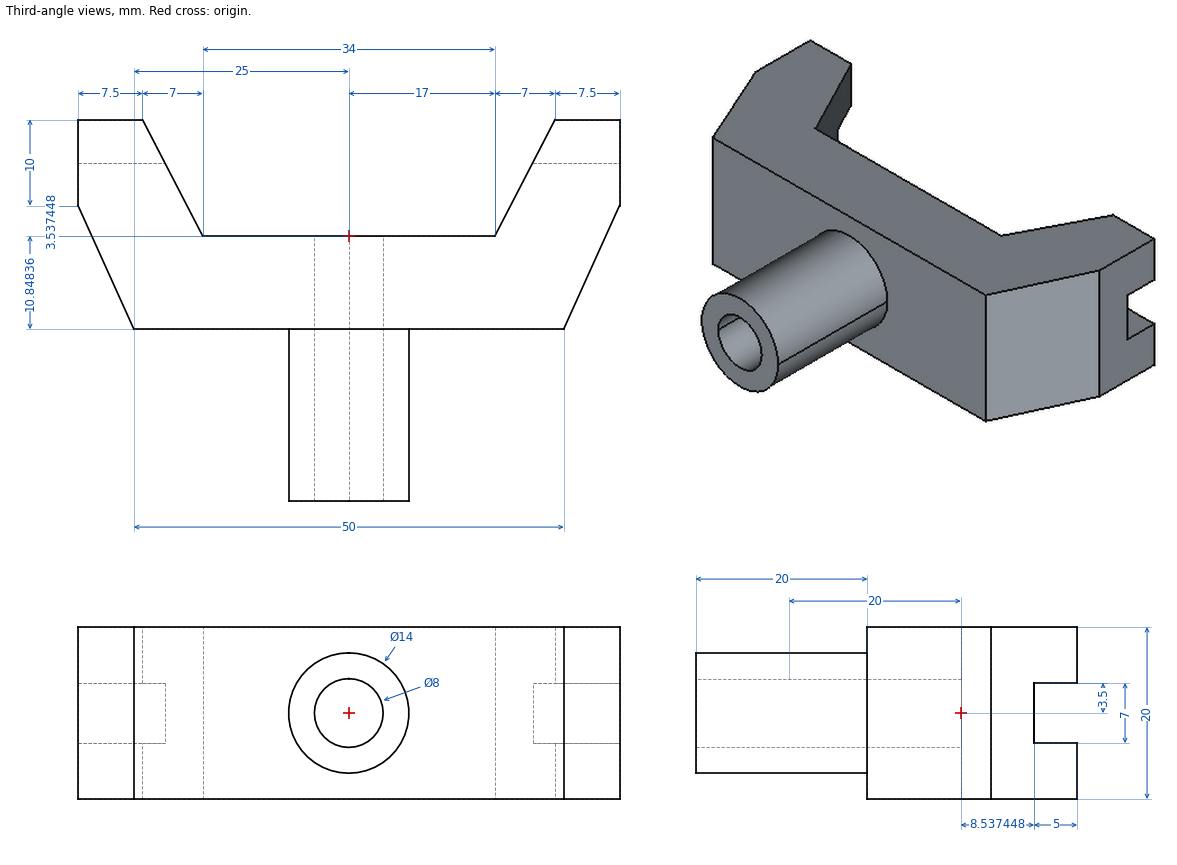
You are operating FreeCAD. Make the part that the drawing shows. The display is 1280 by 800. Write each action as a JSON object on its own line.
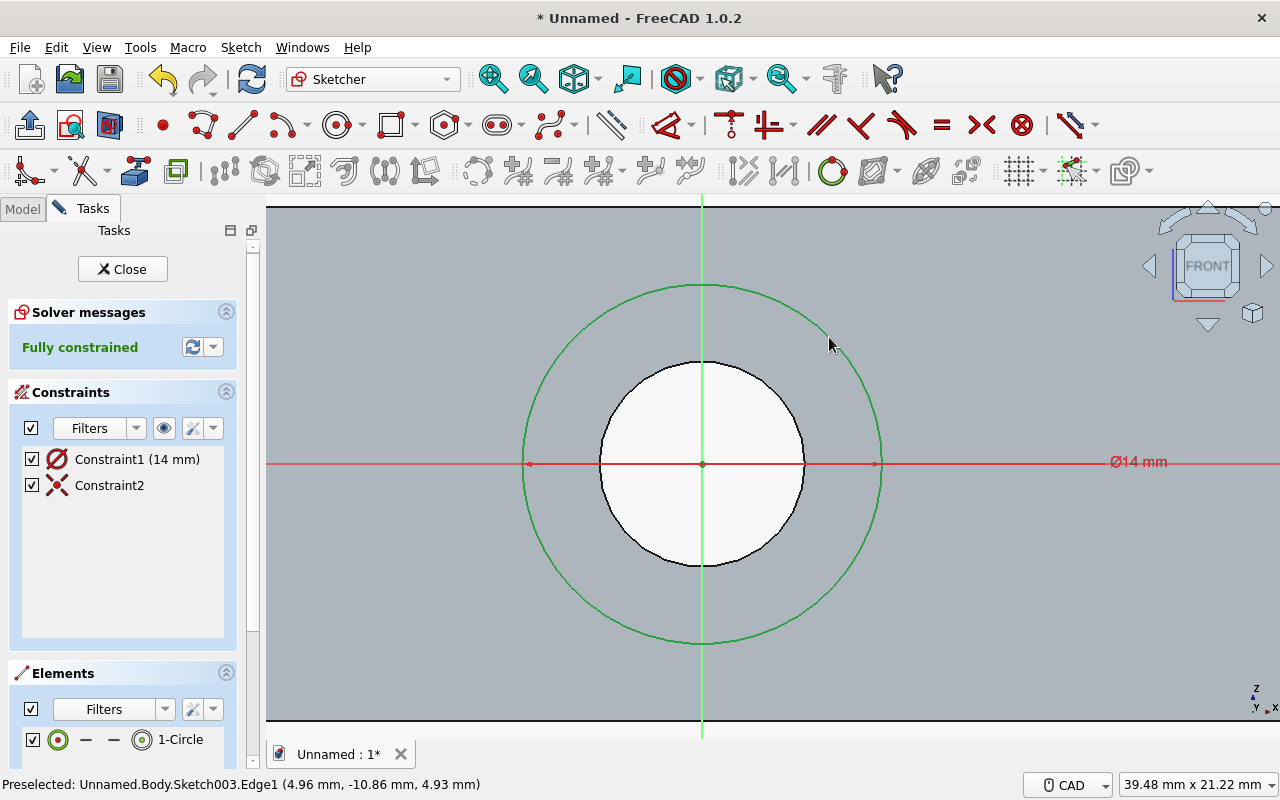
{"action": "left_click", "coordinate": [123, 269]}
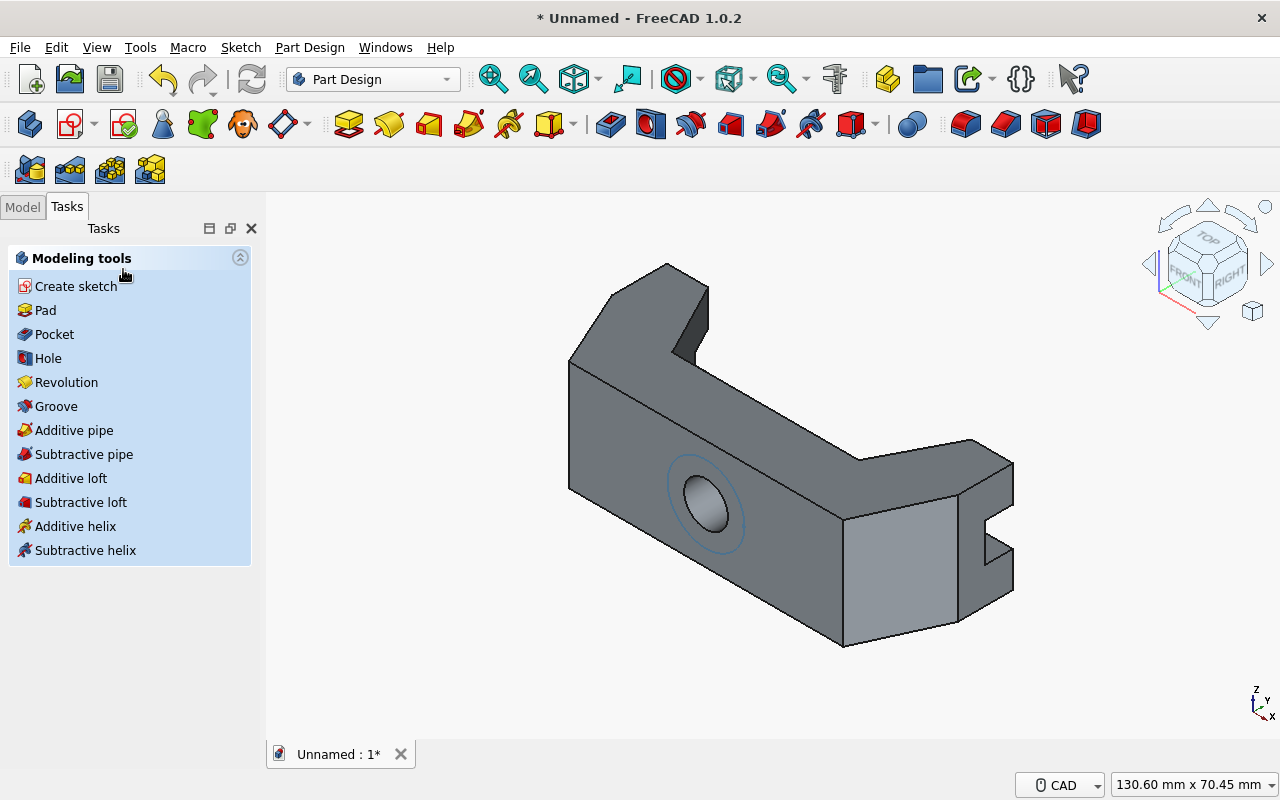
{"action": "left_click", "coordinate": [350, 124]}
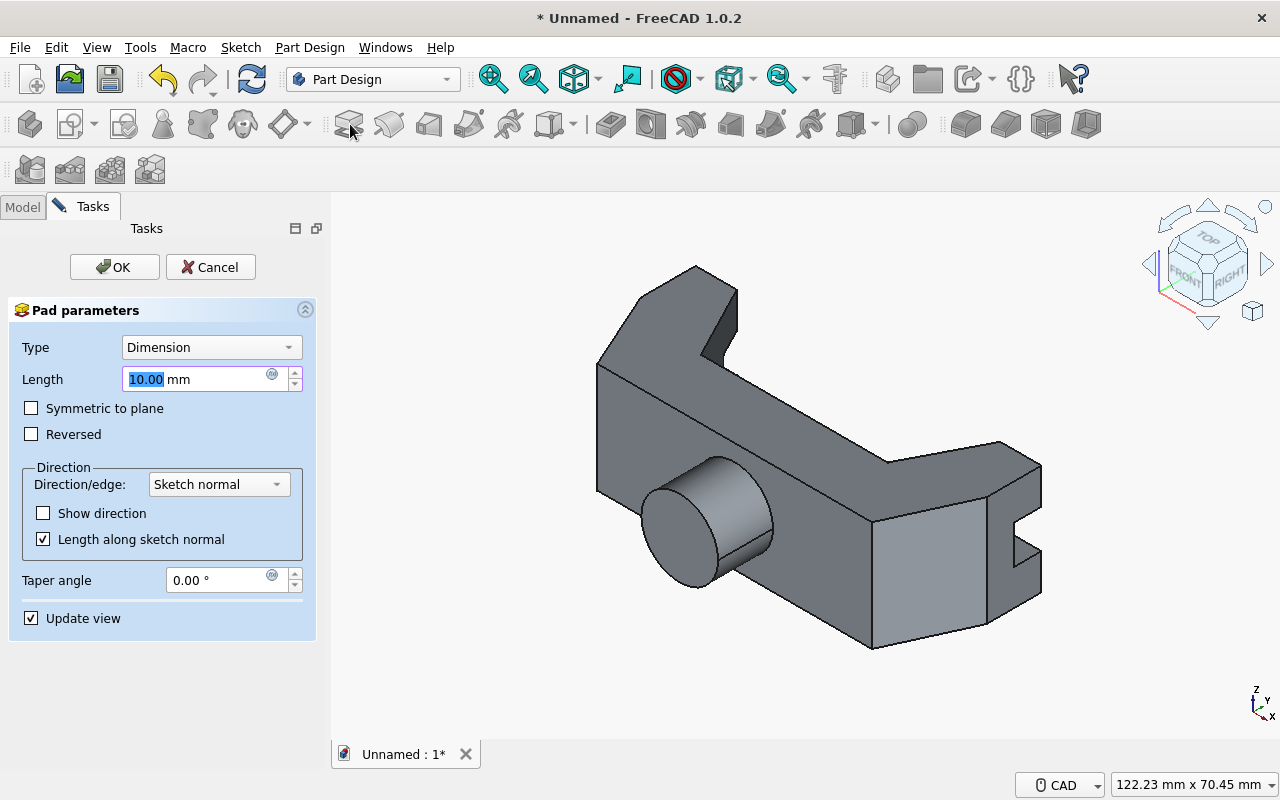
{"action": "type", "text": "20"}
{"action": "key", "text": "Tab"}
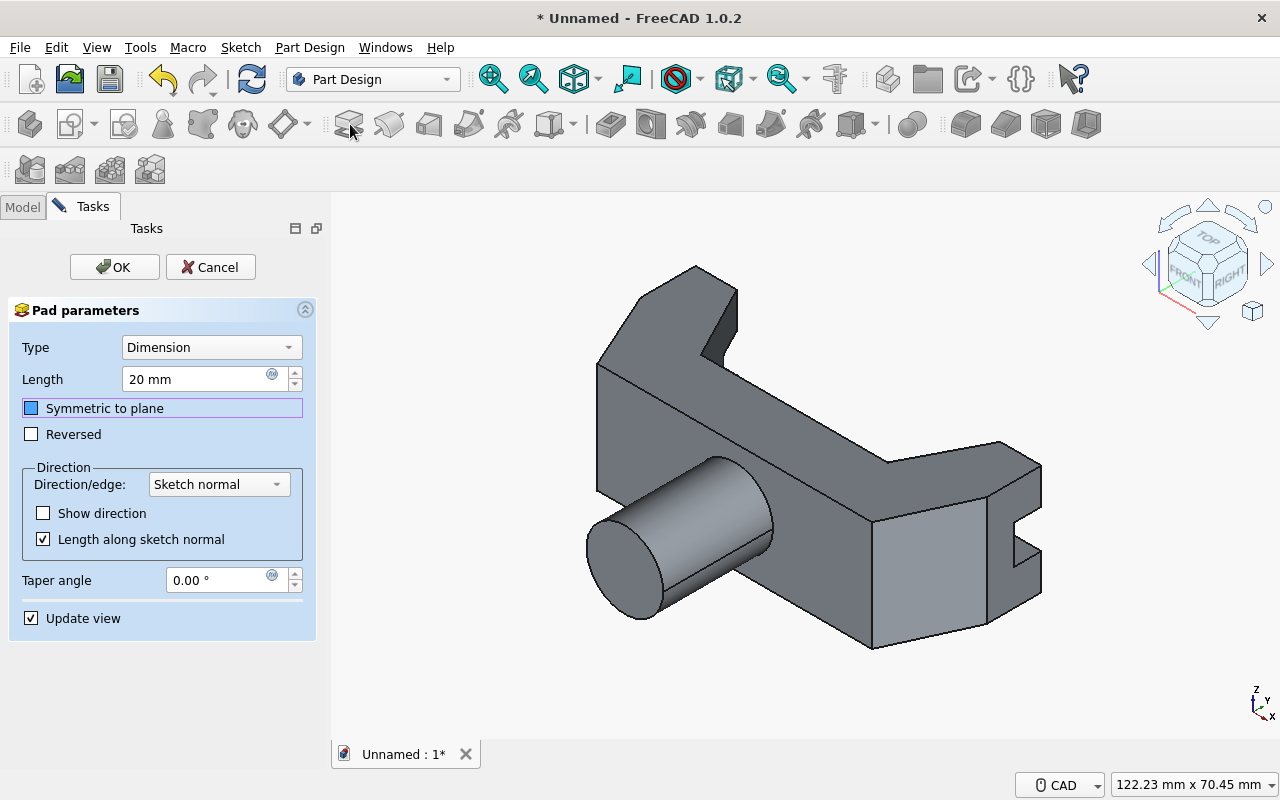
{"action": "left_click", "coordinate": [115, 267]}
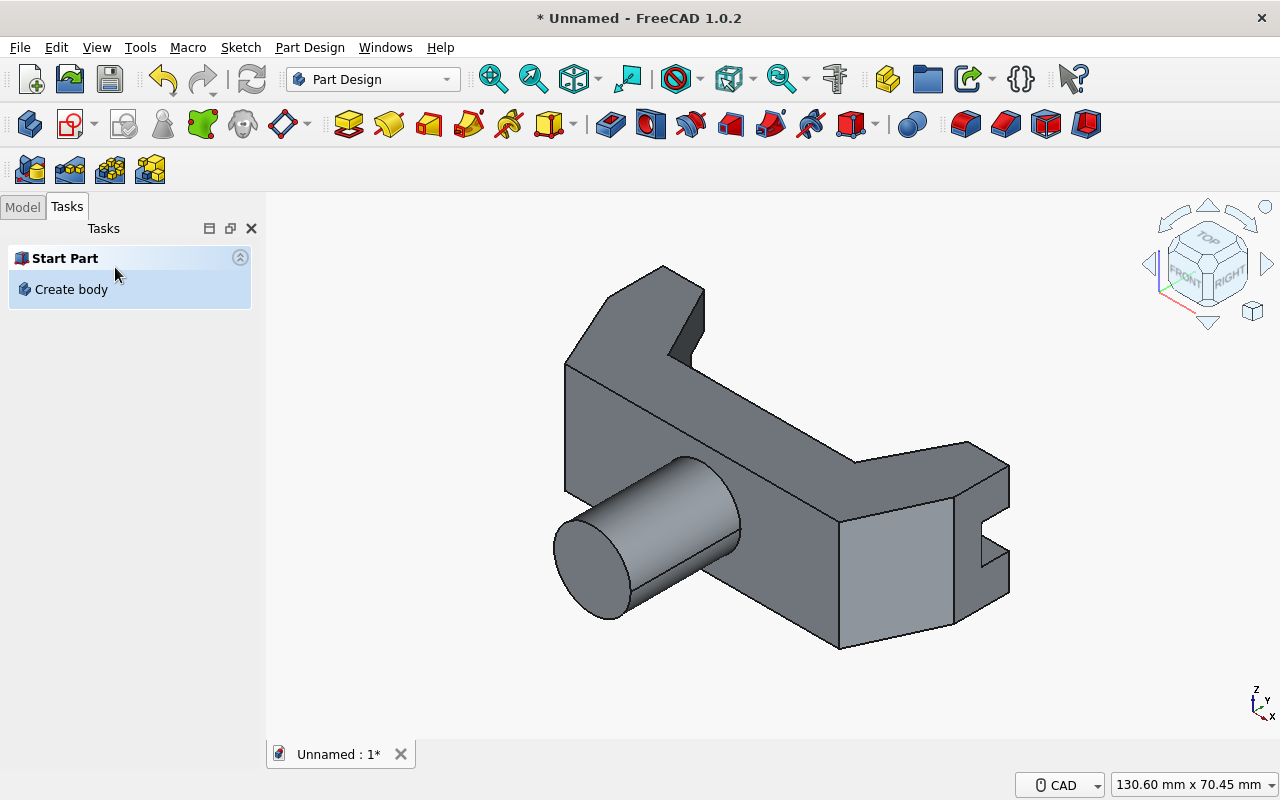
{"action": "key", "text": "4"}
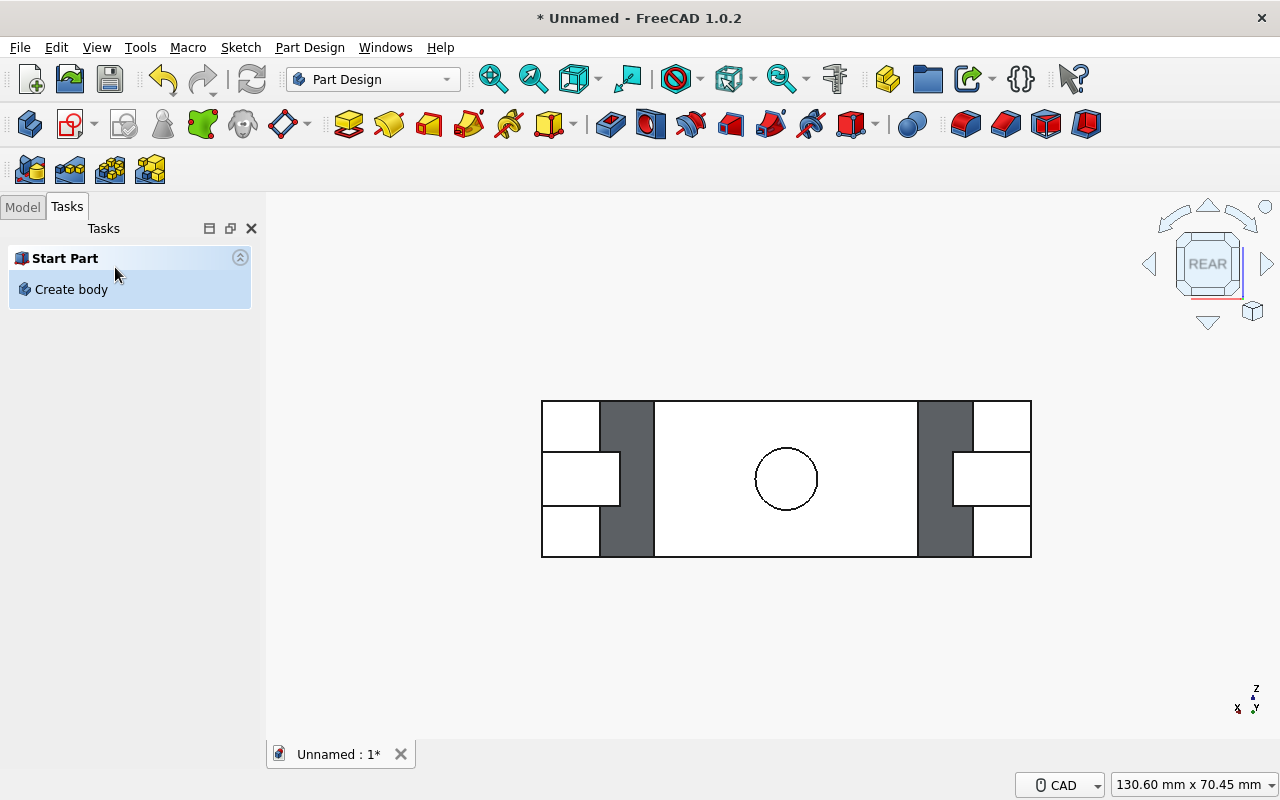
{"action": "left_click", "coordinate": [711, 500]}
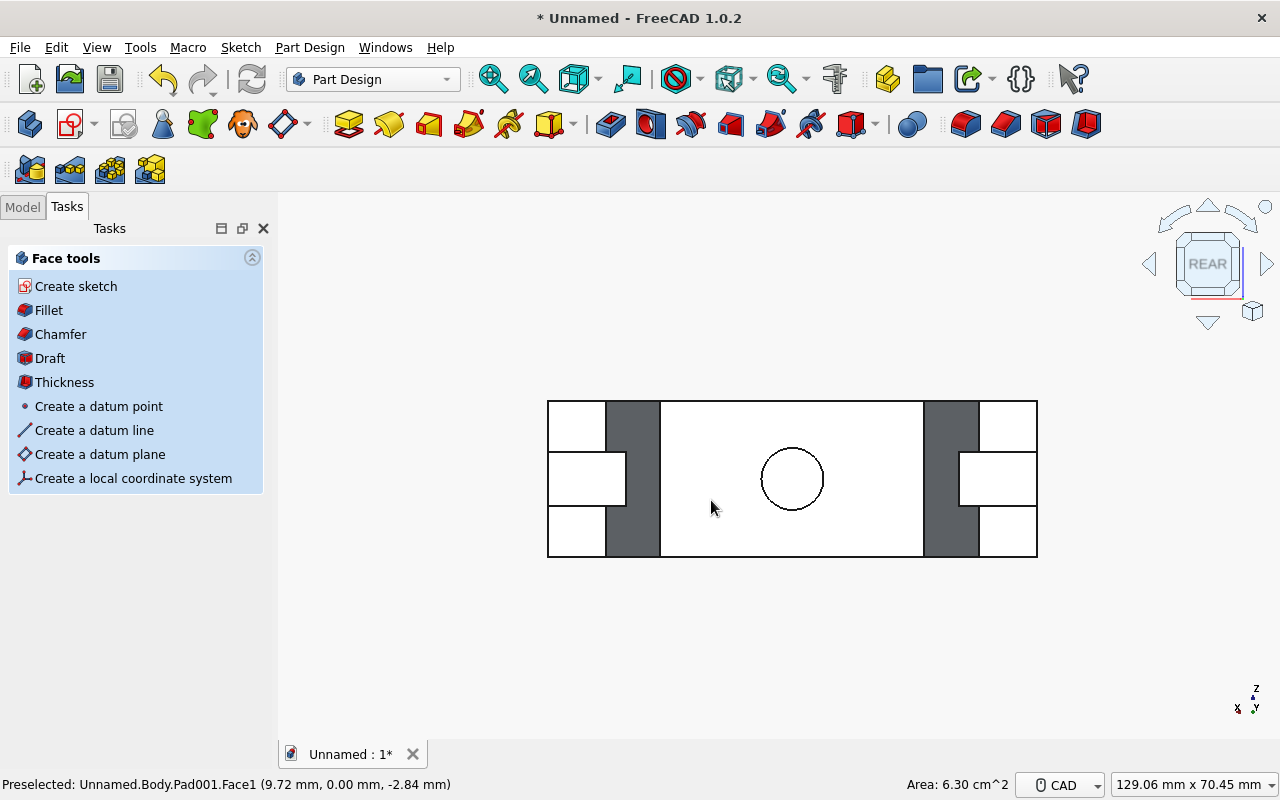
{"action": "left_click", "coordinate": [70, 124]}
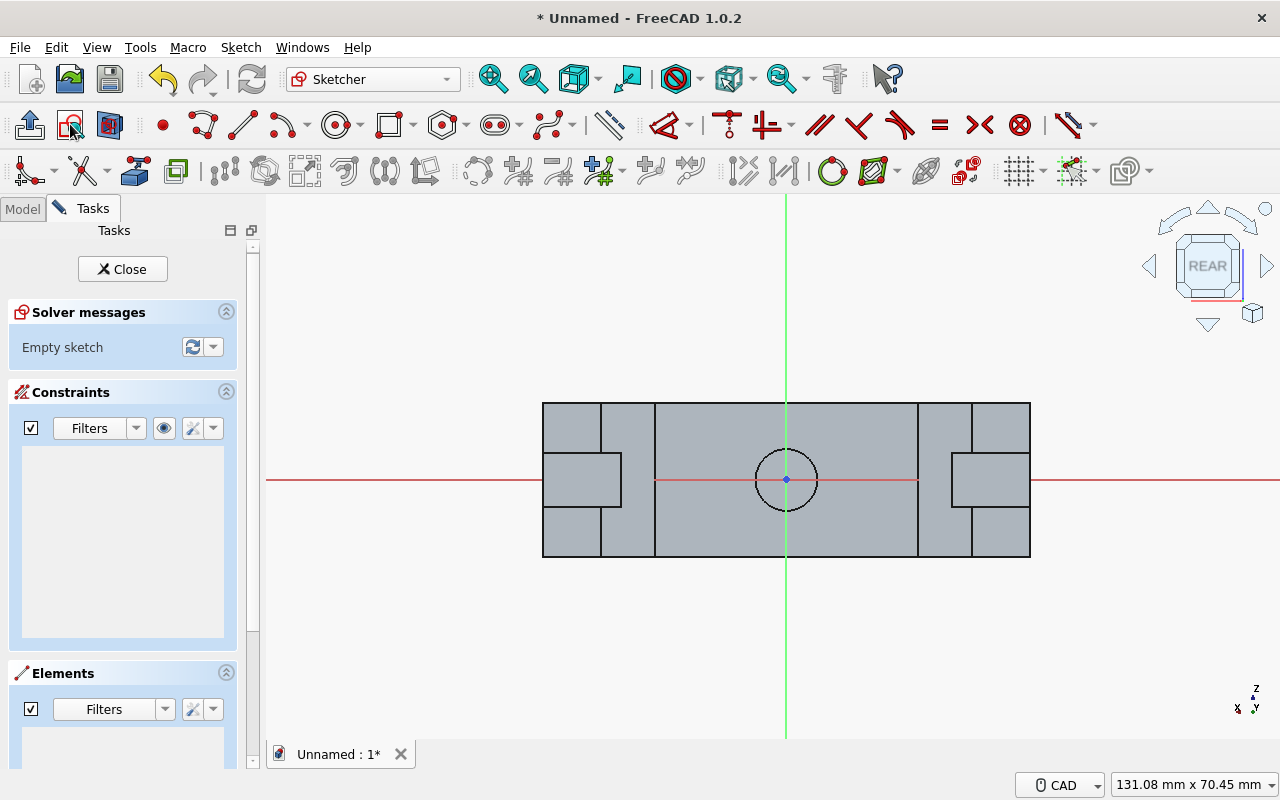
{"action": "left_click", "coordinate": [110, 126]}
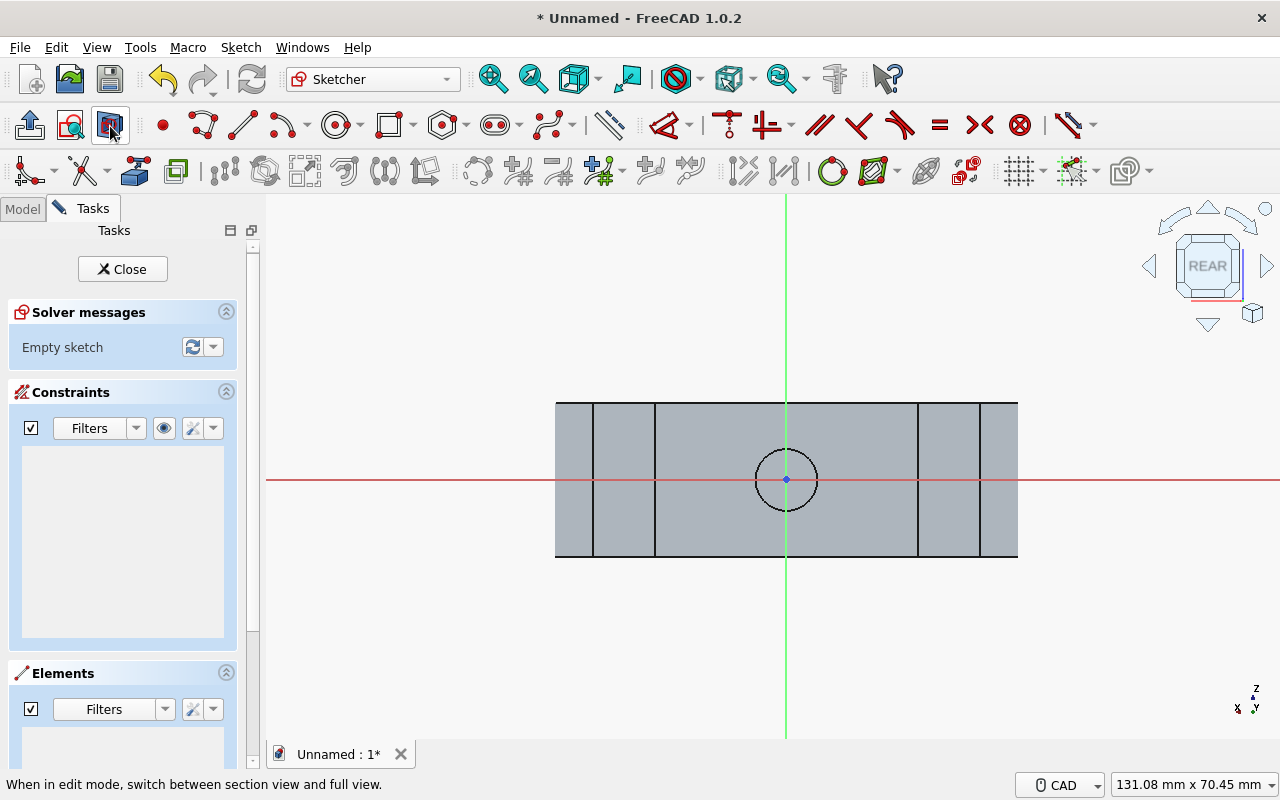
{"action": "scroll", "coordinate": [803, 483], "scroll_direction": "up", "scroll_amount": 9}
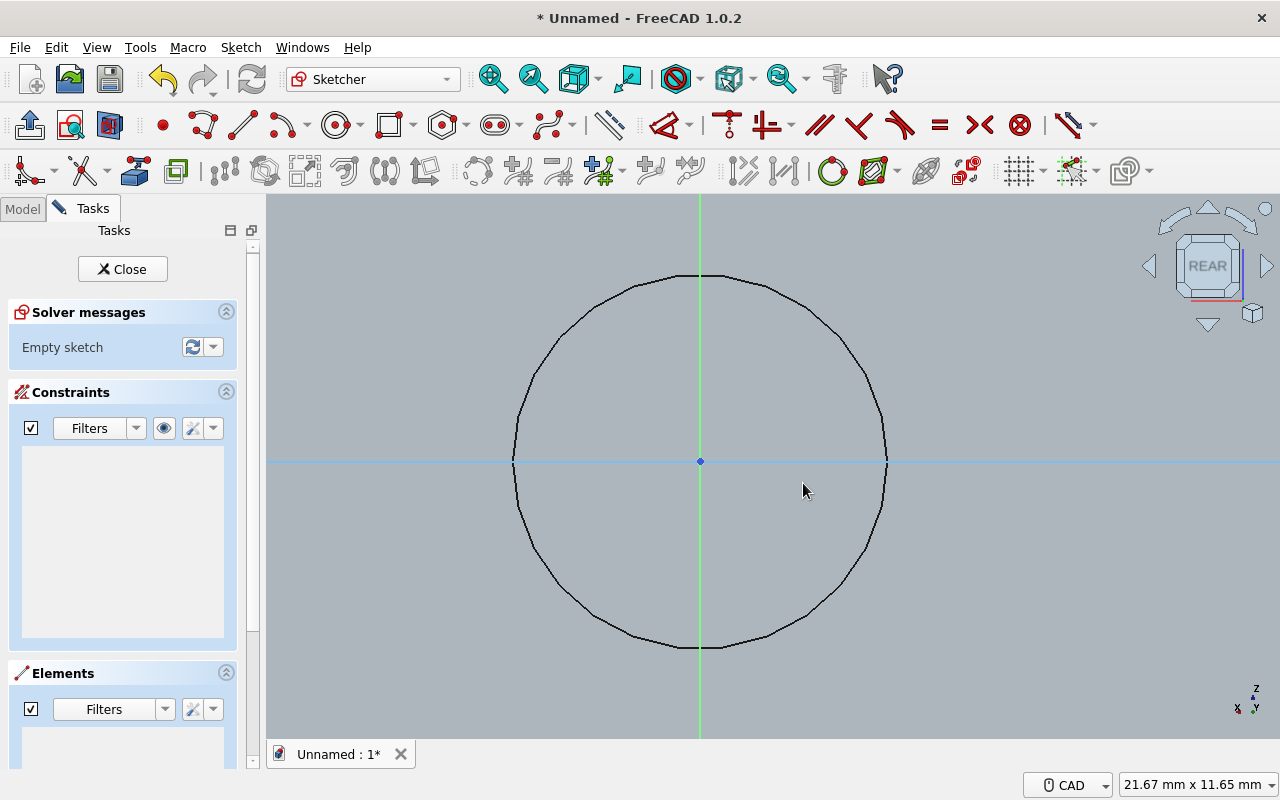
{"action": "left_click", "coordinate": [336, 126]}